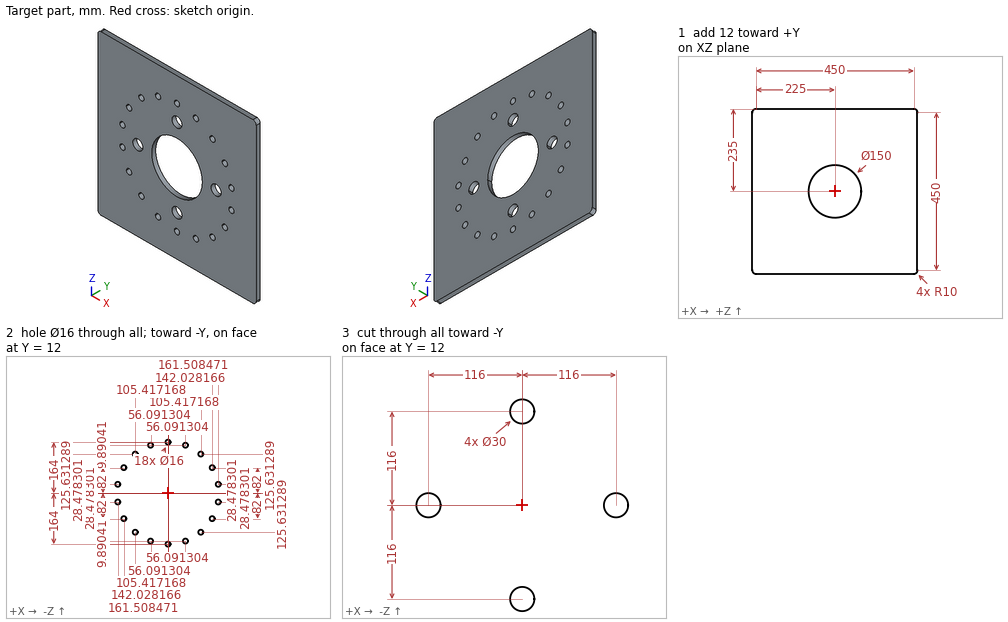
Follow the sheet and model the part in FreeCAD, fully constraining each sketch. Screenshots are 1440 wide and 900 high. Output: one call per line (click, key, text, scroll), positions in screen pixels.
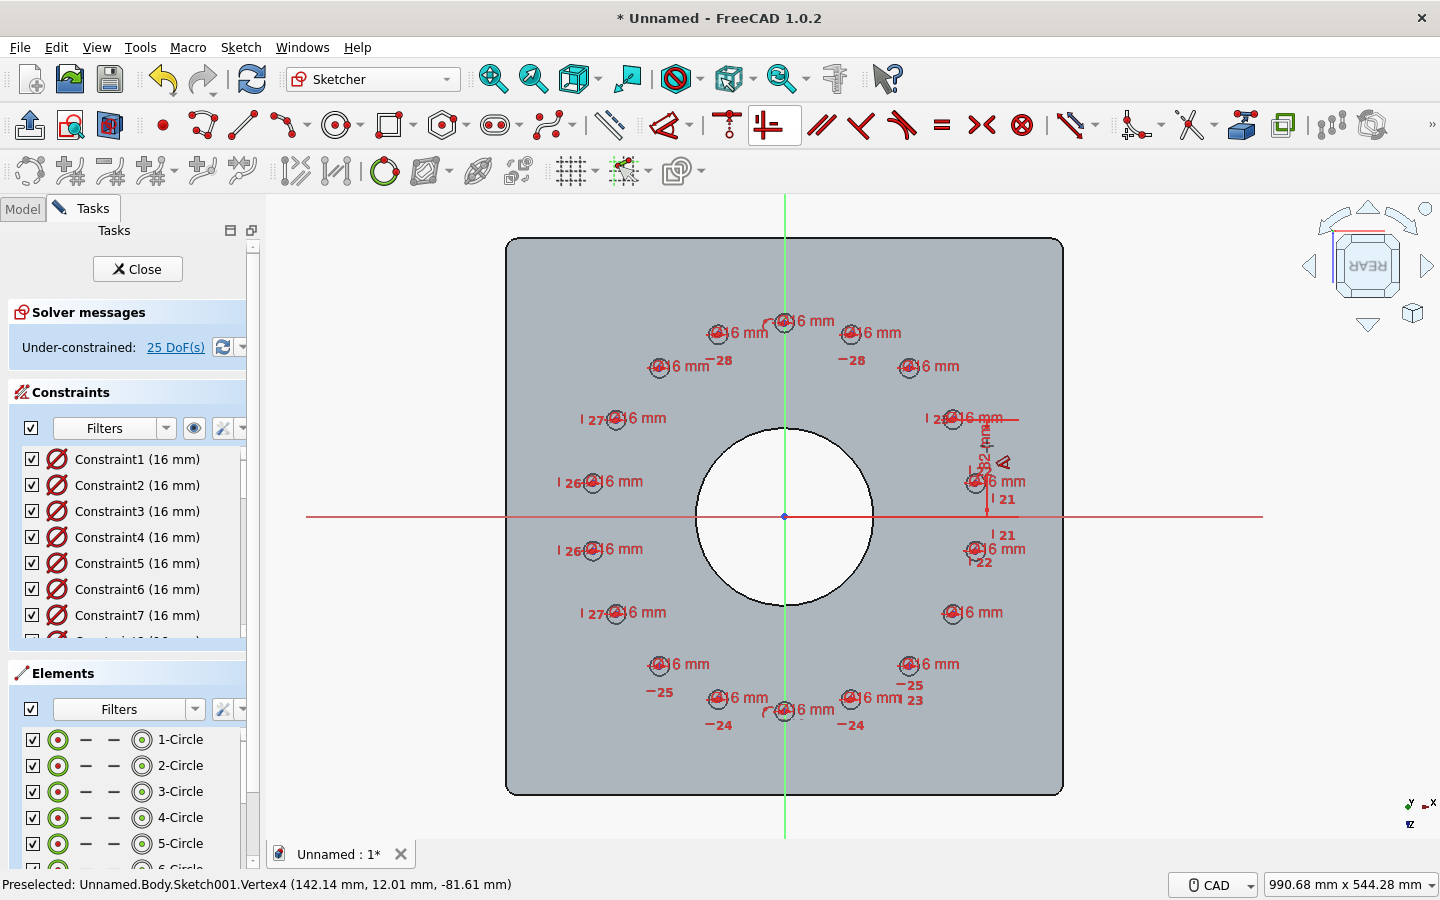
click(953, 614)
click(987, 588)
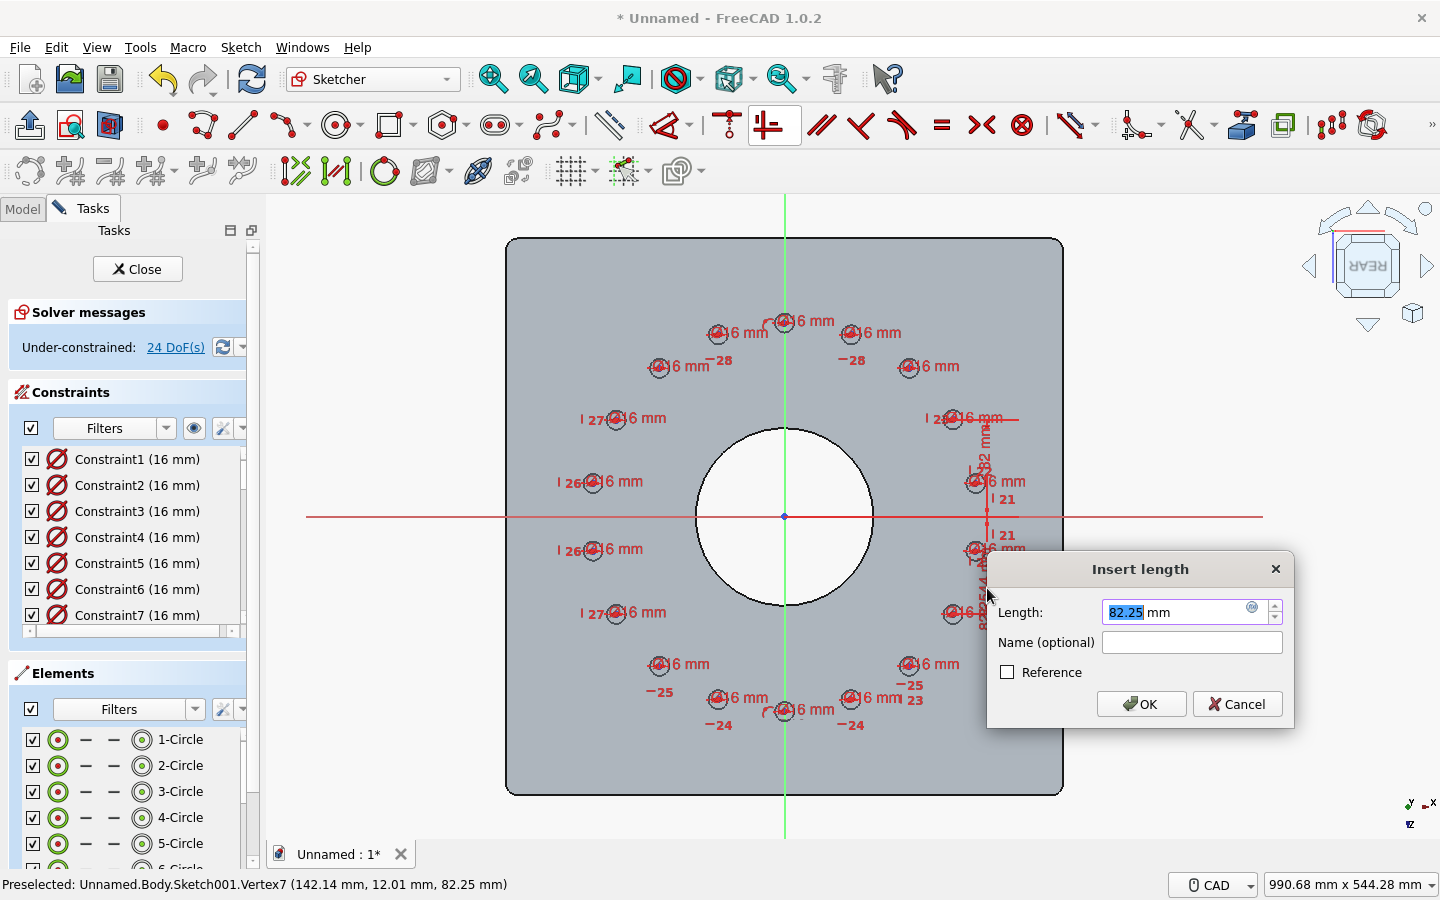
text(82)
key(Return)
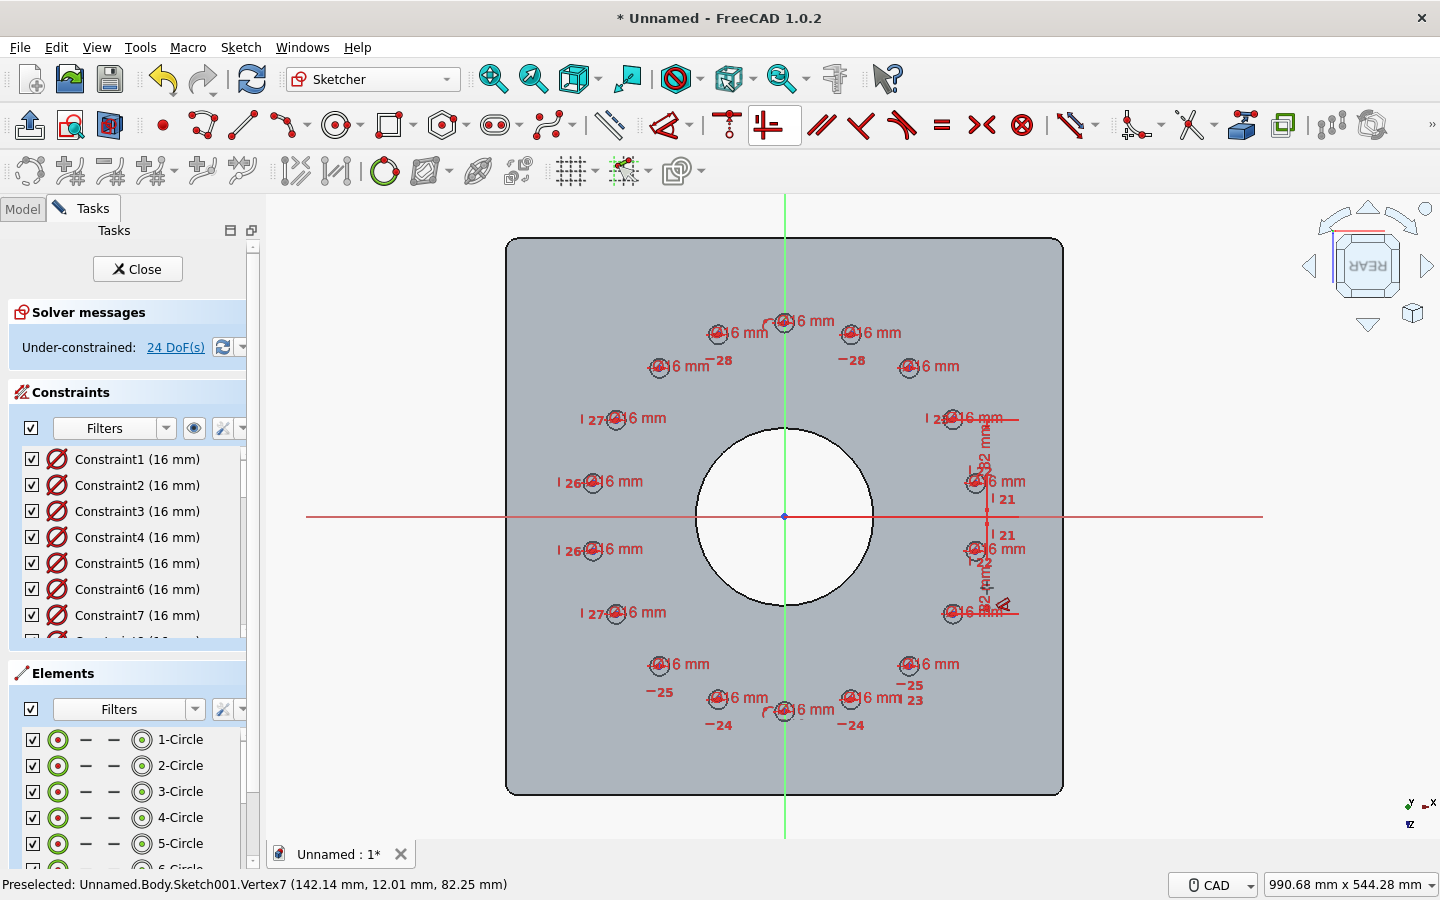
click(616, 614)
click(582, 588)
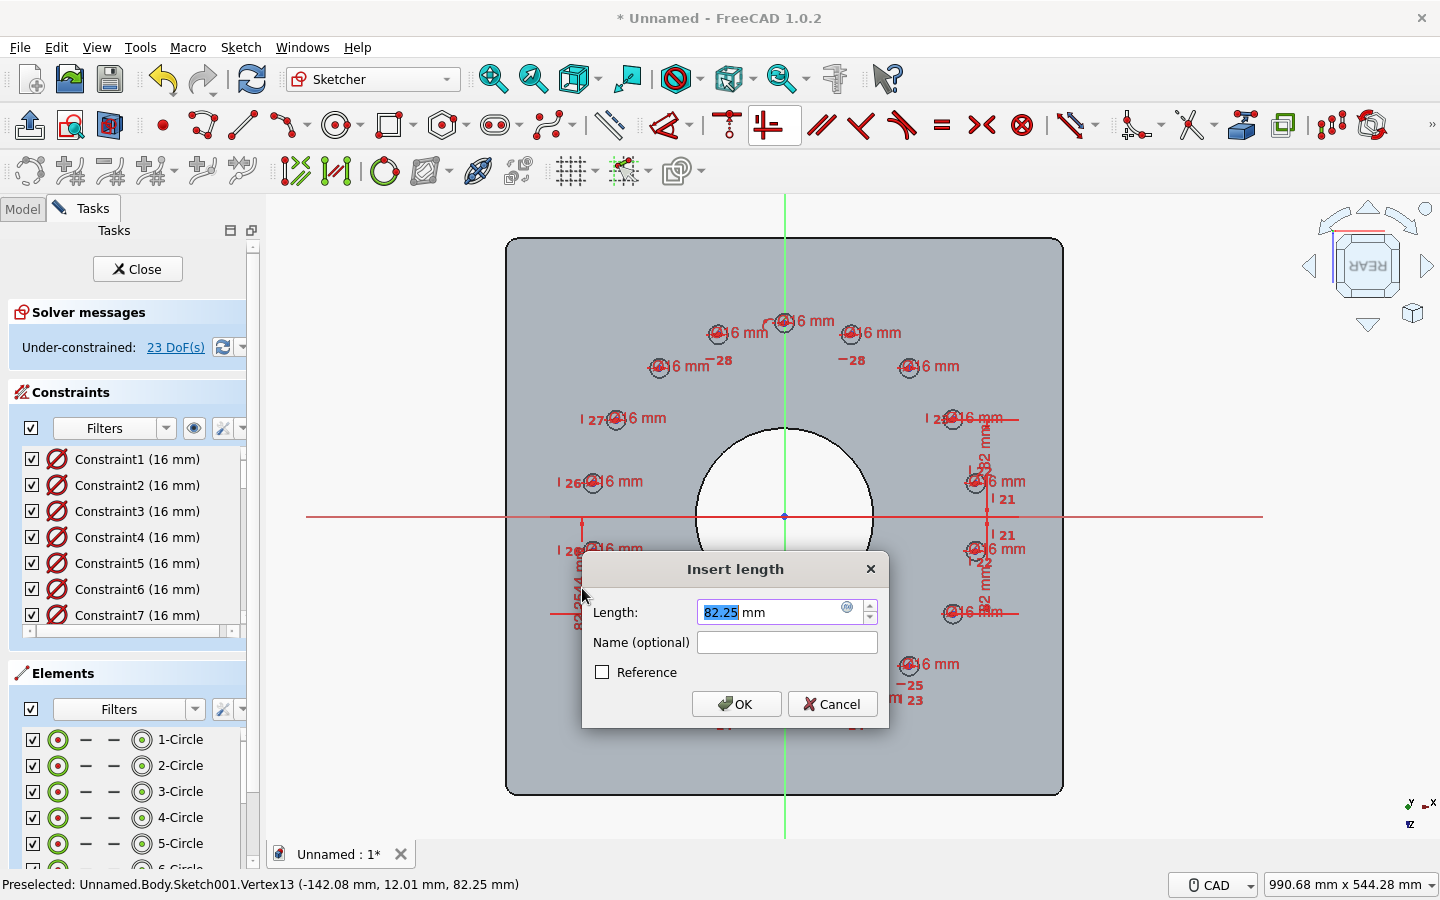
text(82)
key(Return)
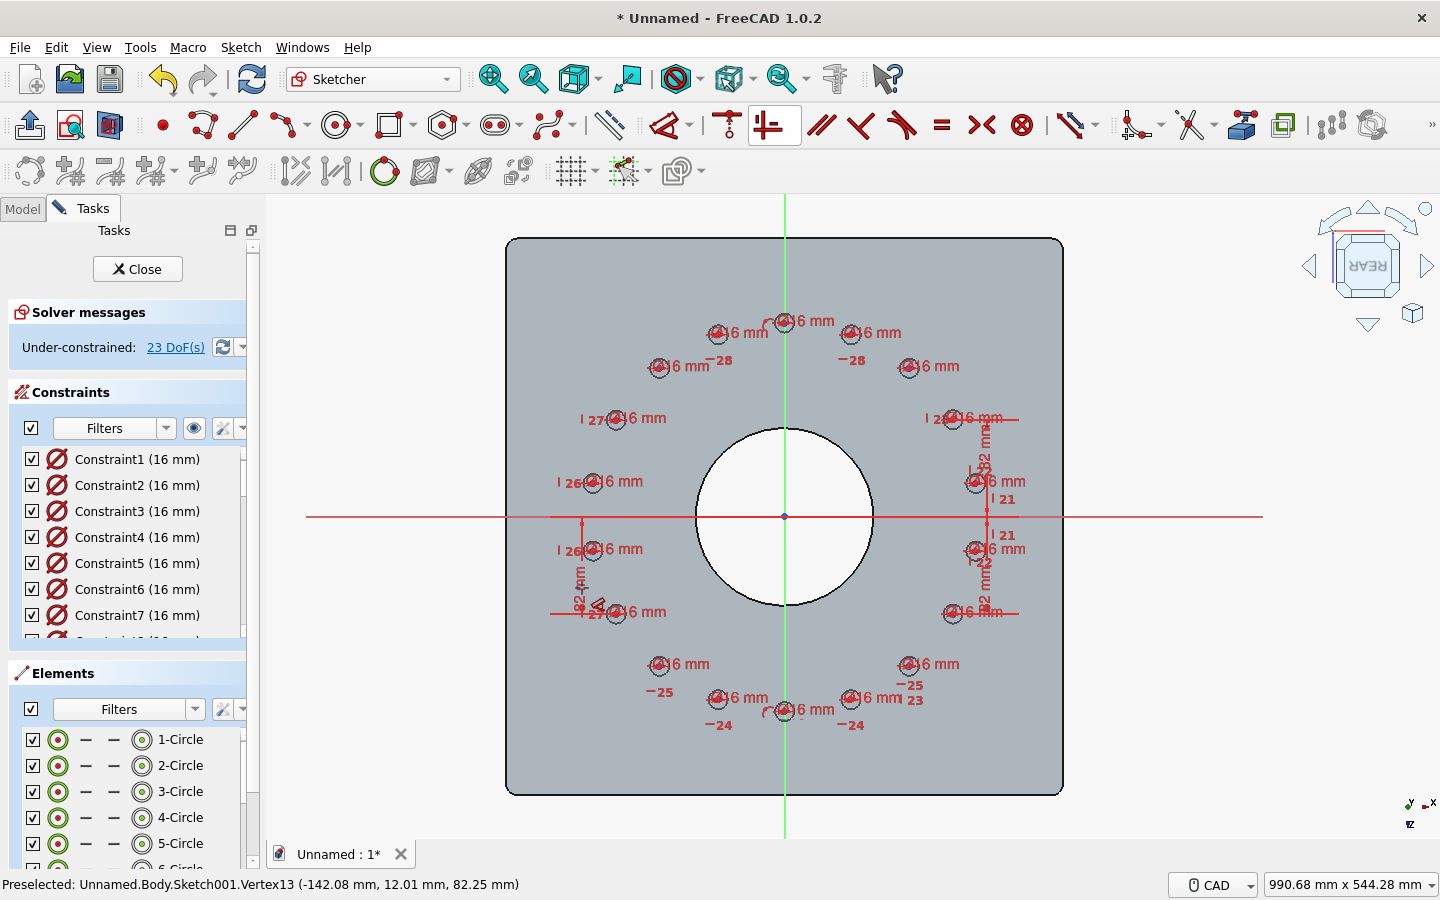
click(616, 420)
click(582, 446)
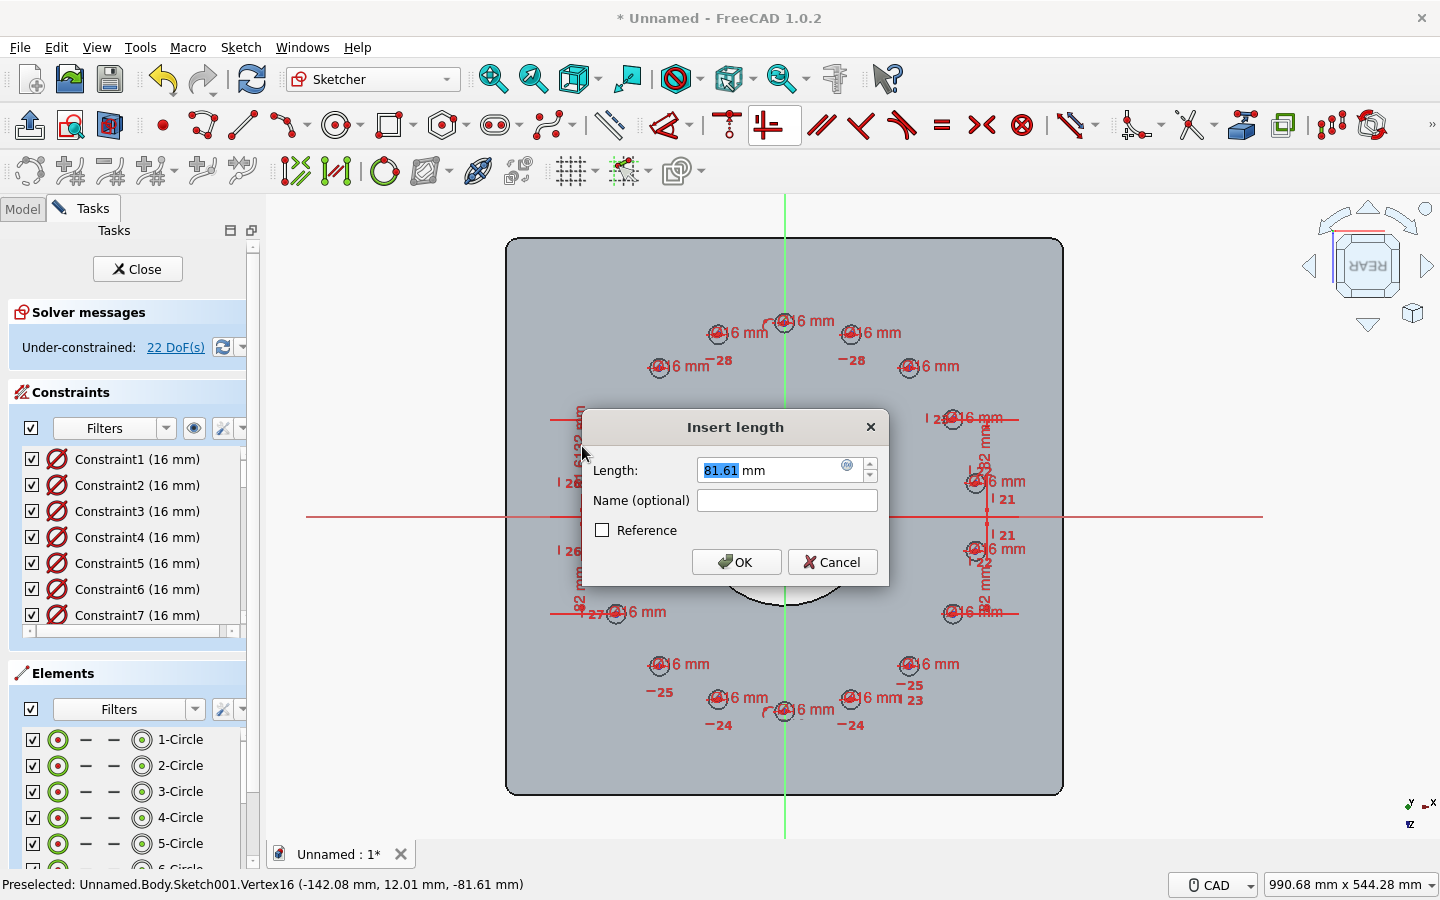
text(82)
key(Return)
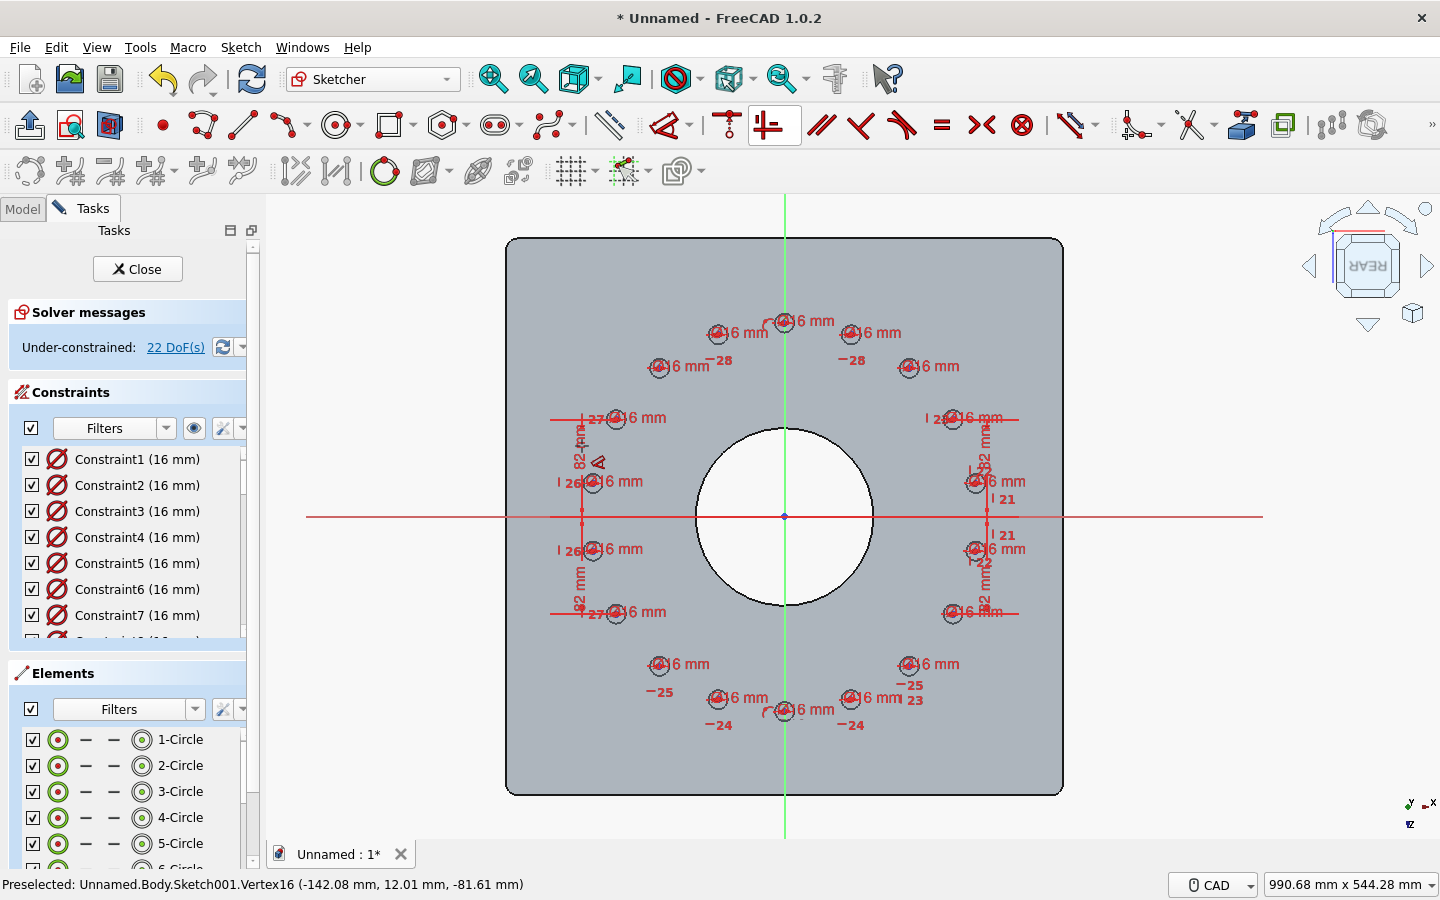
click(785, 323)
click(819, 420)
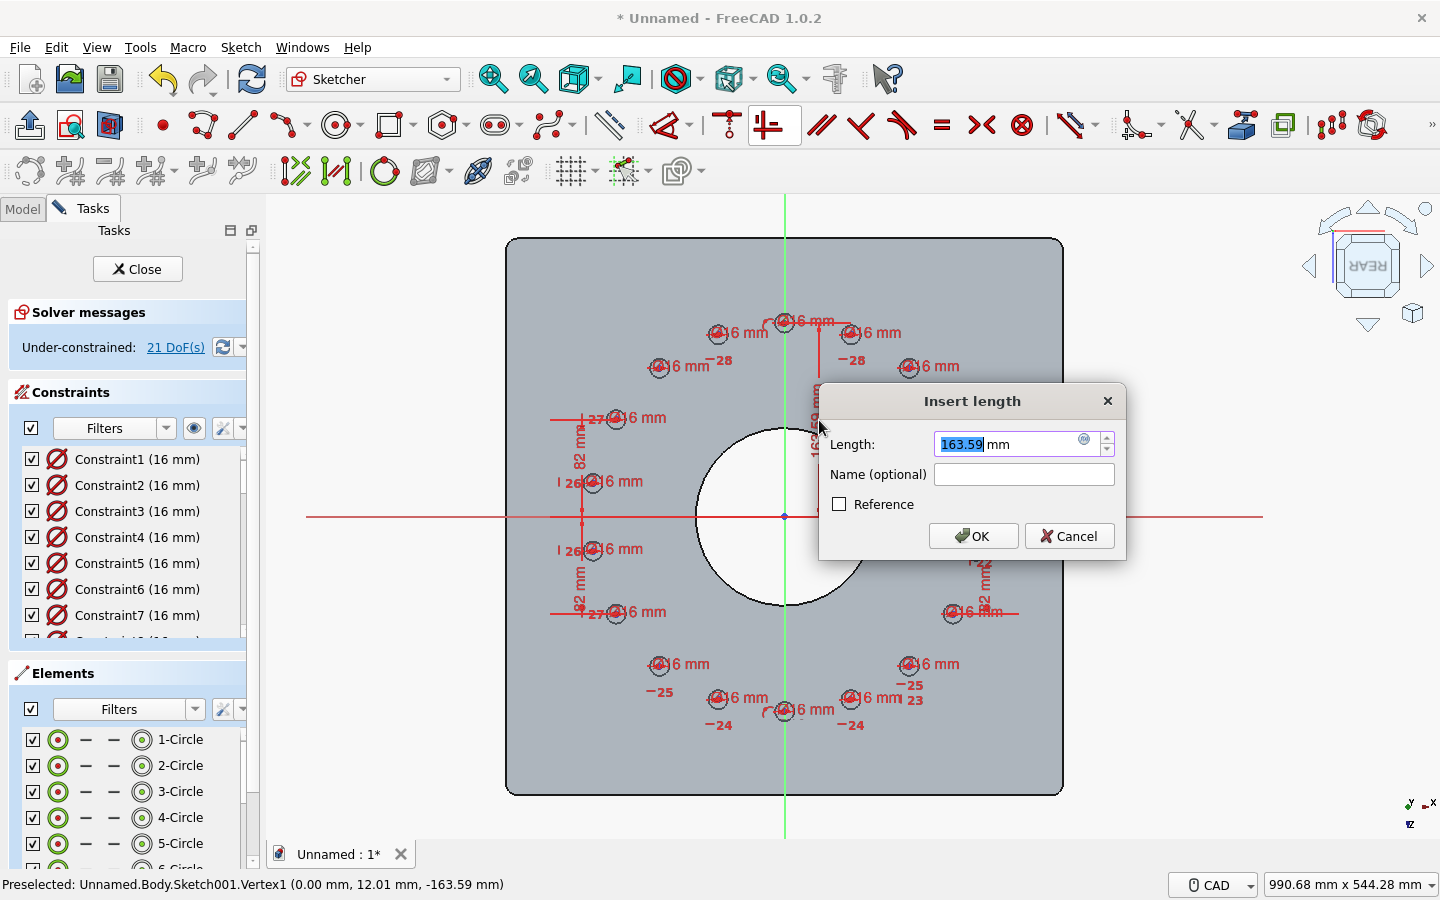
text(164)
key(Return)